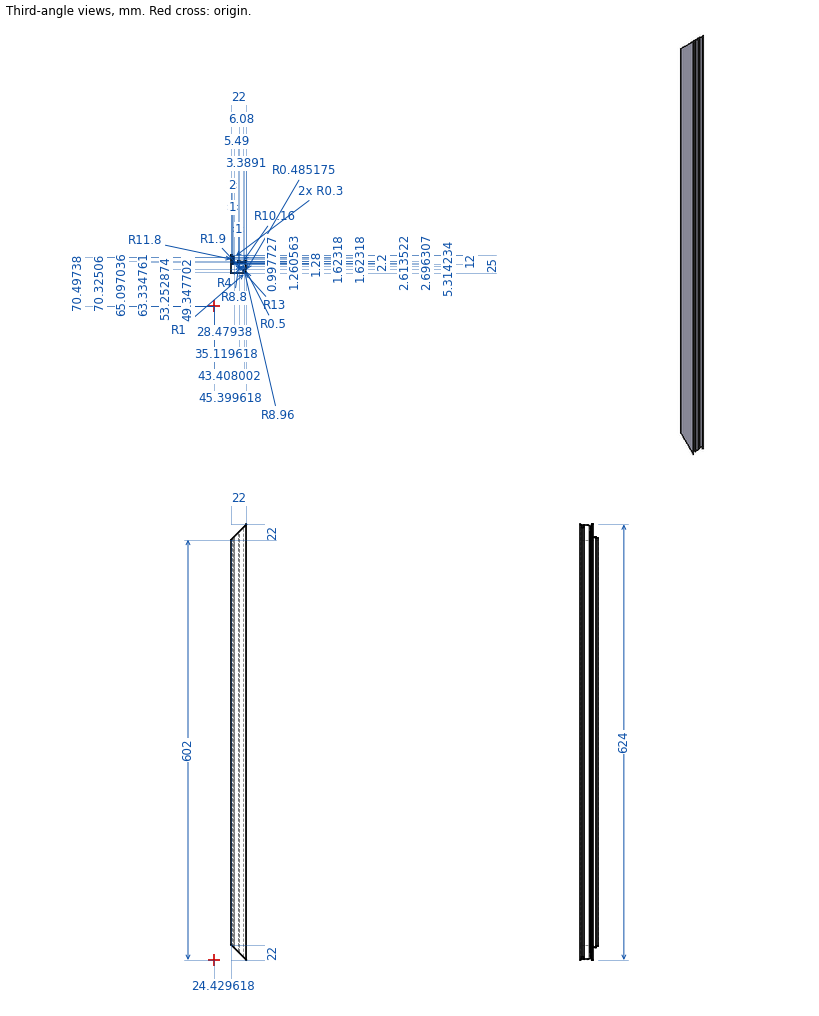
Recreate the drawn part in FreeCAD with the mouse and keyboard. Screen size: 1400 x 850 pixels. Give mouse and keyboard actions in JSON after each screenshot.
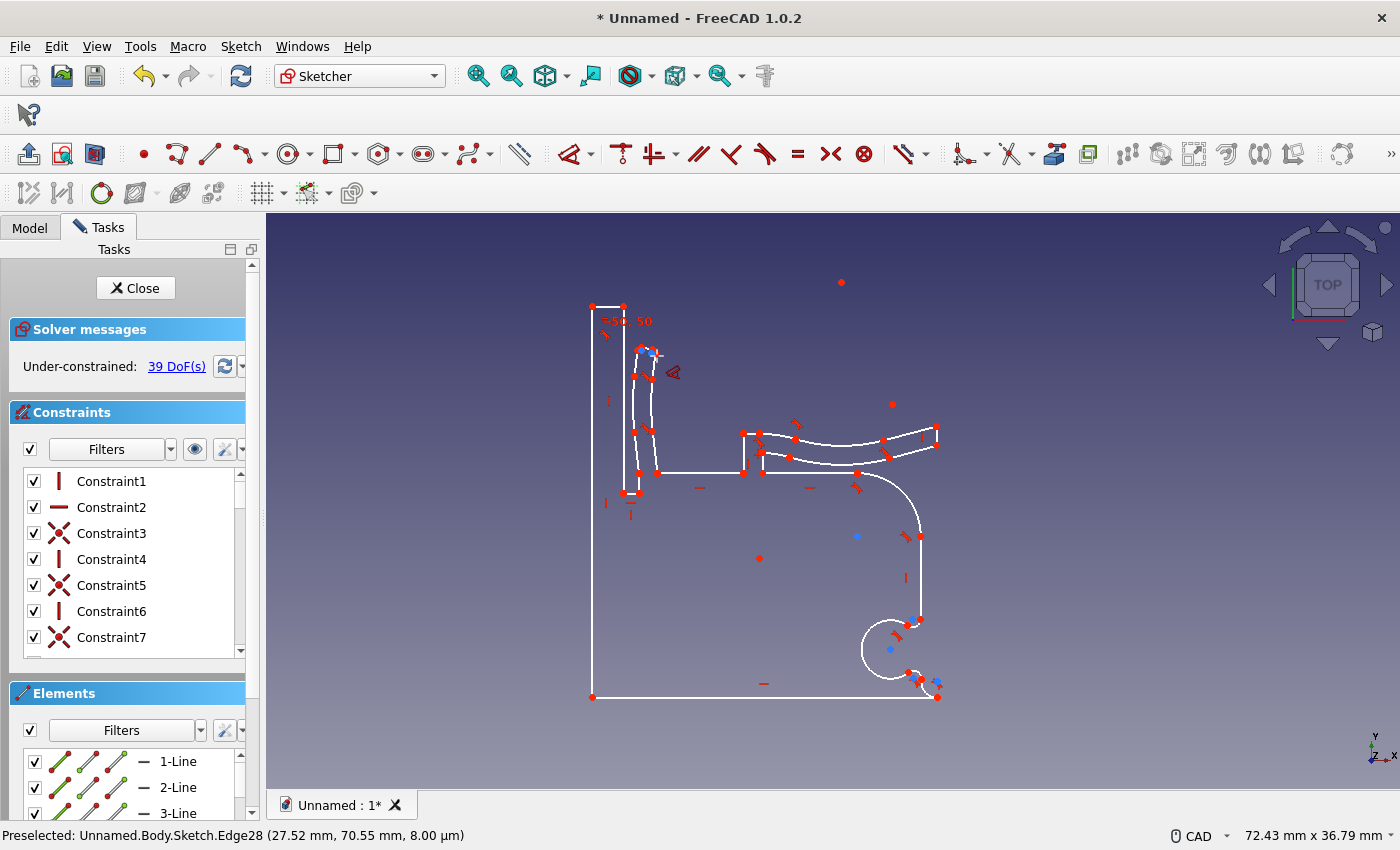
{"action": "left_click", "coordinate": [914, 508]}
{"action": "left_click", "coordinate": [943, 494]}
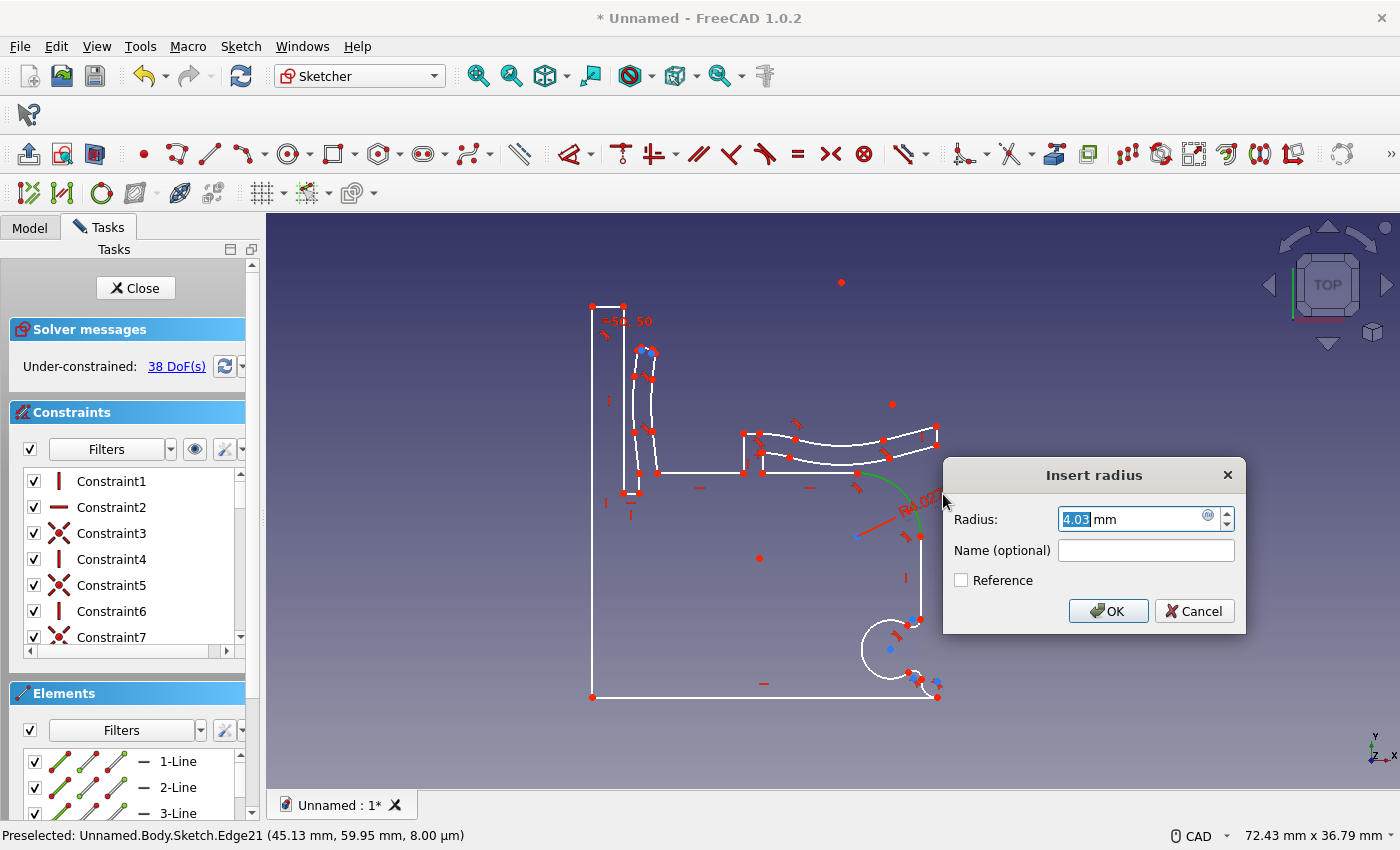
{"action": "type", "text": "4"}
{"action": "key", "text": "Return"}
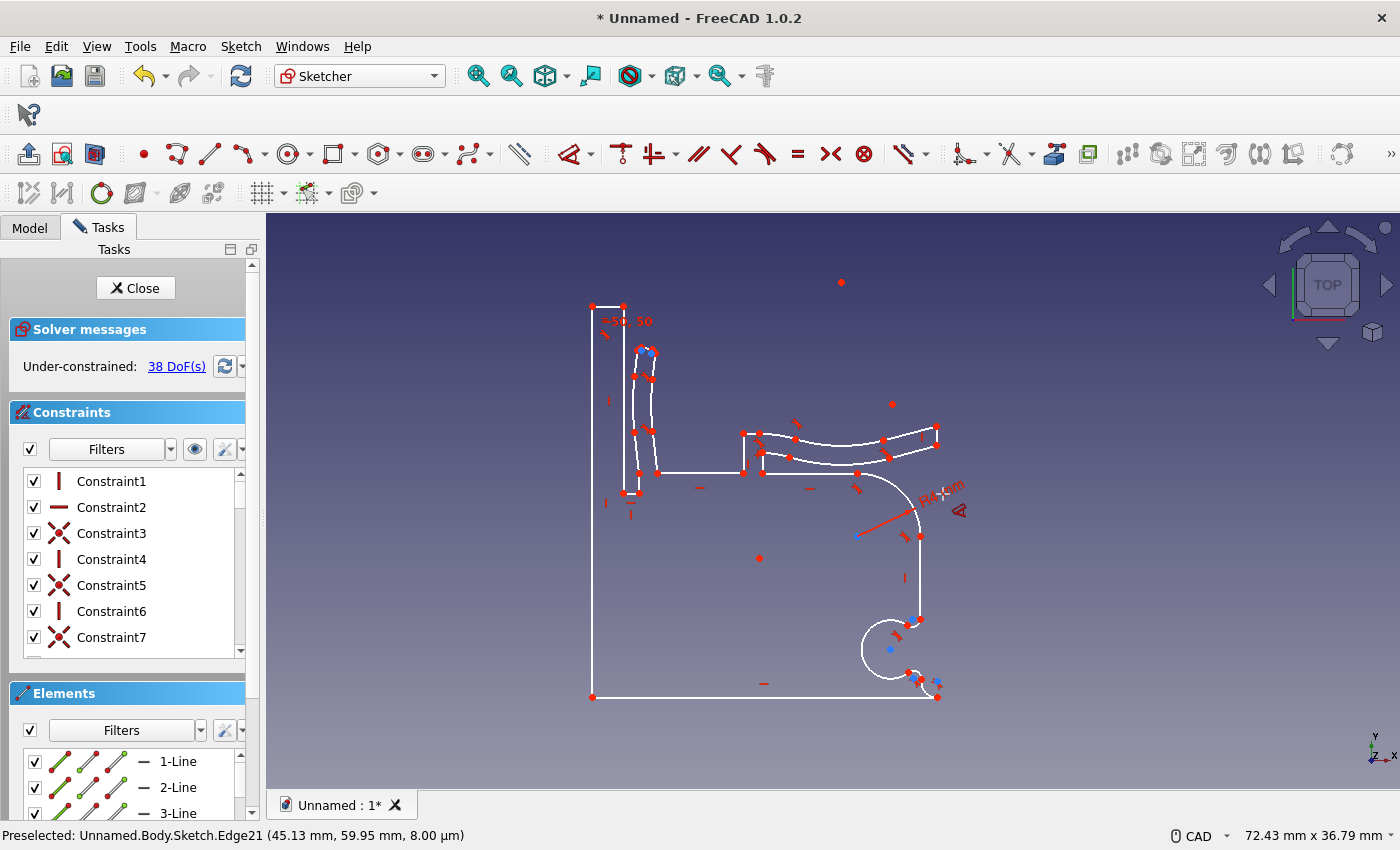
{"action": "left_click", "coordinate": [776, 454]}
{"action": "left_click", "coordinate": [781, 422]}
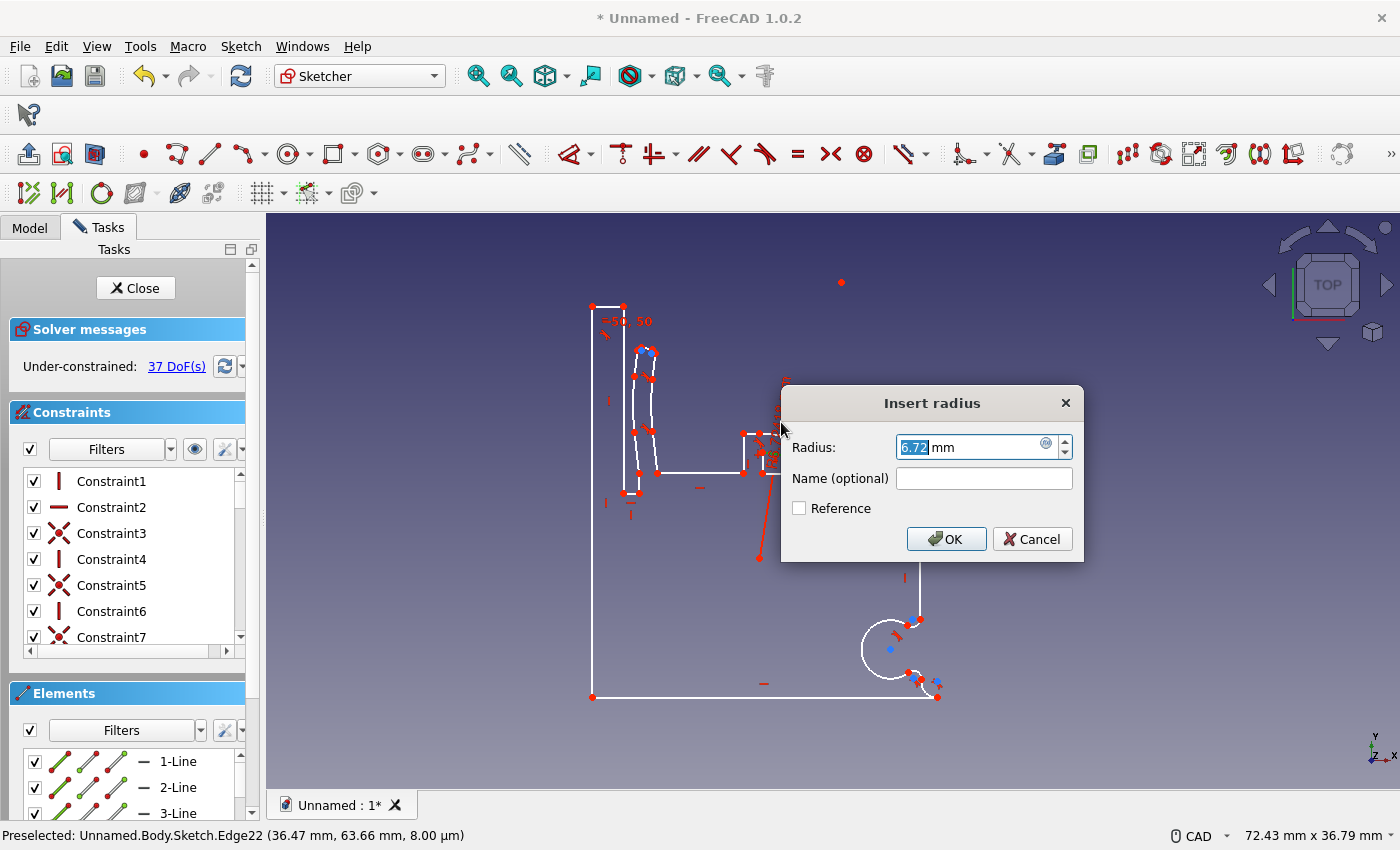
{"action": "type", "text": "8.8"}
{"action": "key", "text": "Return"}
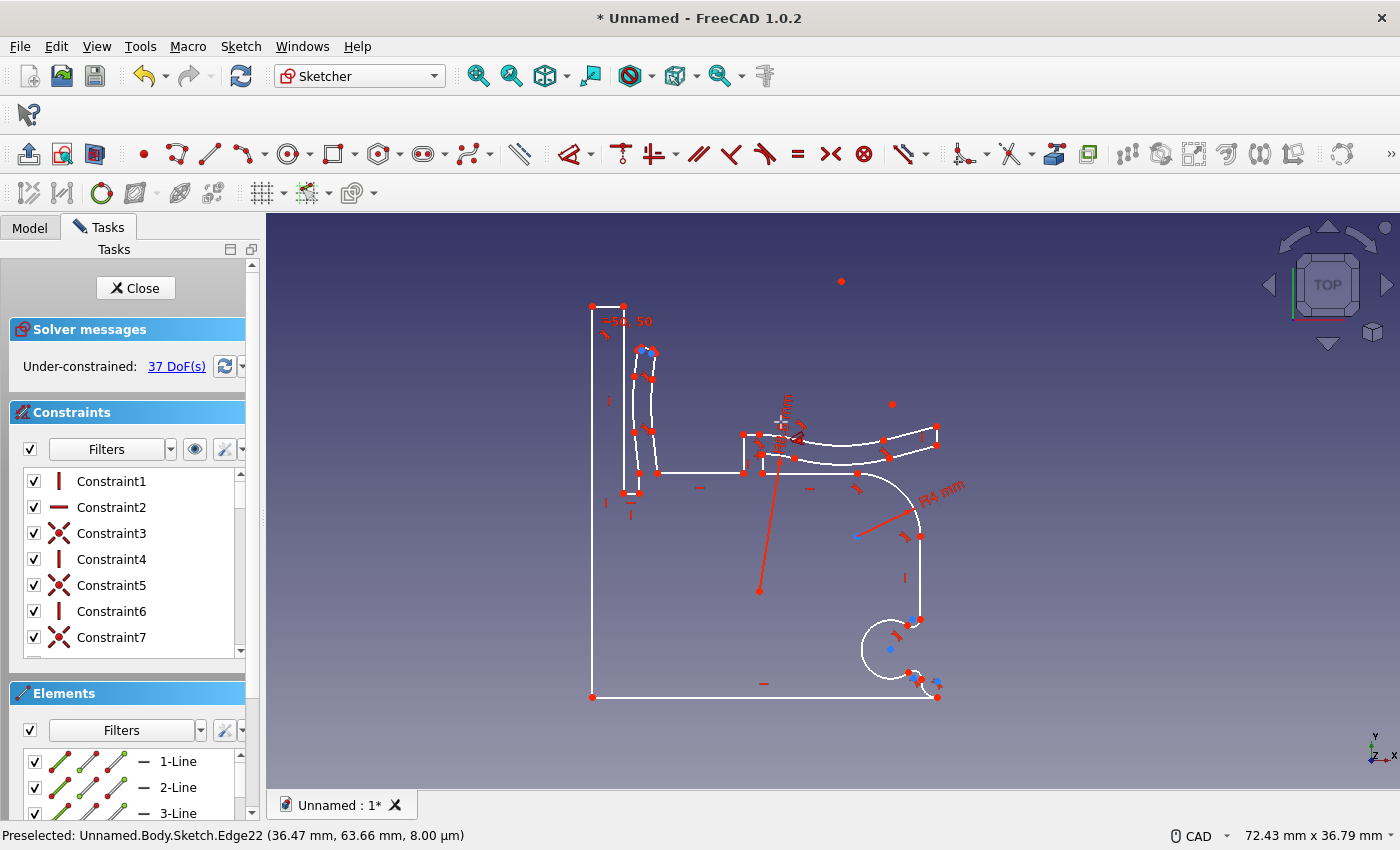
{"action": "scroll", "coordinate": [823, 464], "scroll_direction": "up", "scroll_amount": 2}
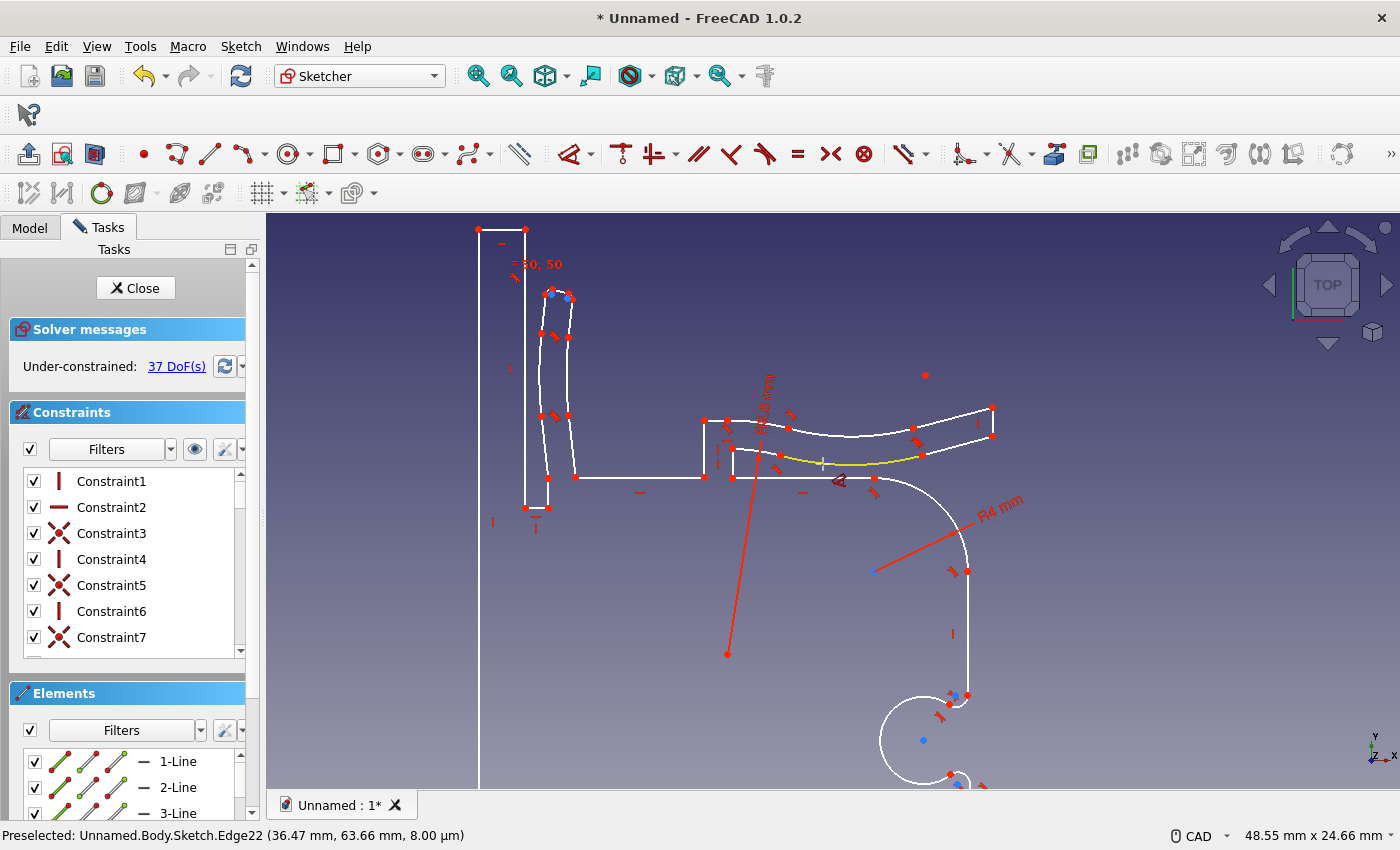
{"action": "left_click", "coordinate": [823, 464]}
{"action": "left_click", "coordinate": [820, 496]}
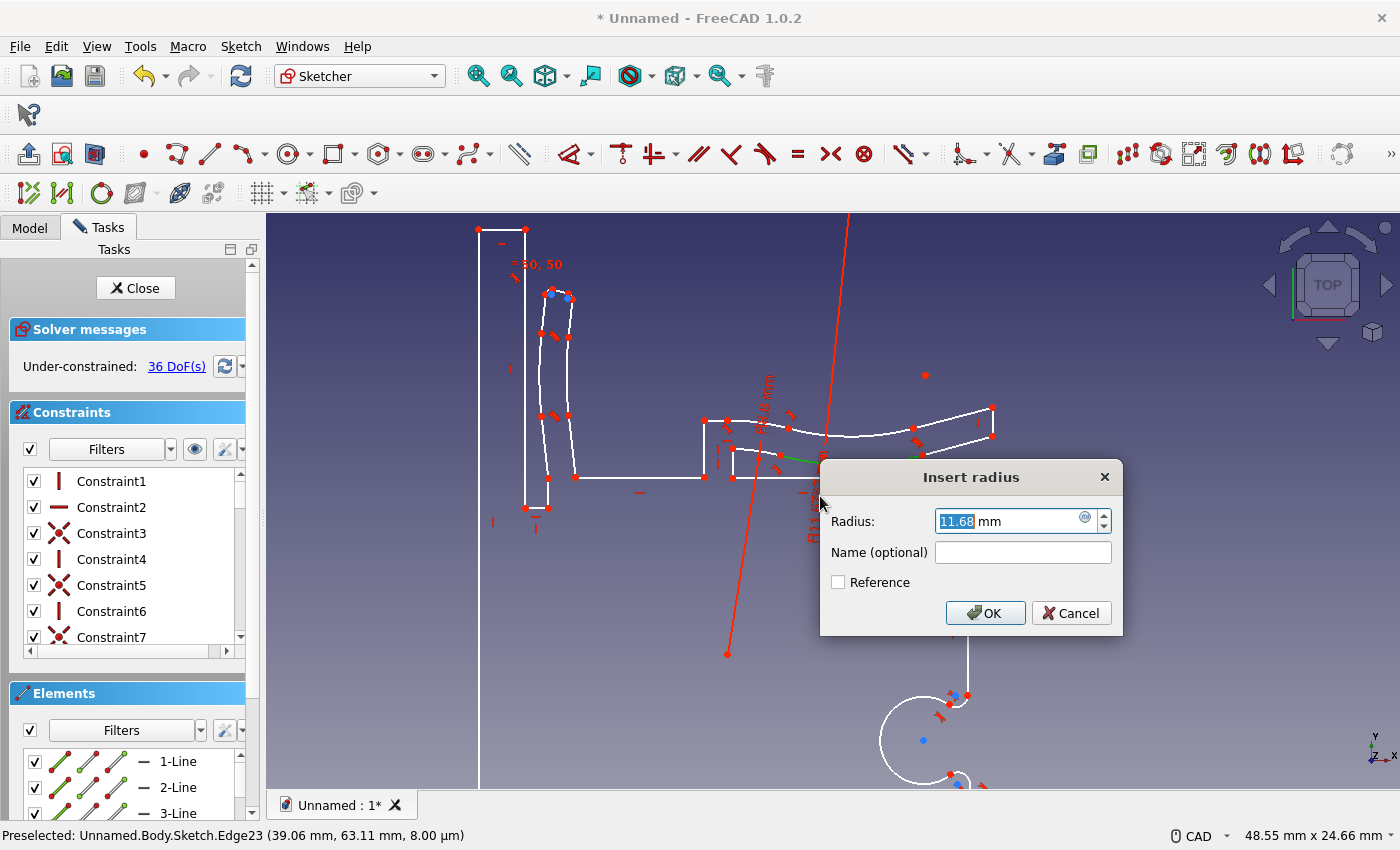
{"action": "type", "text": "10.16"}
{"action": "key", "text": "Return"}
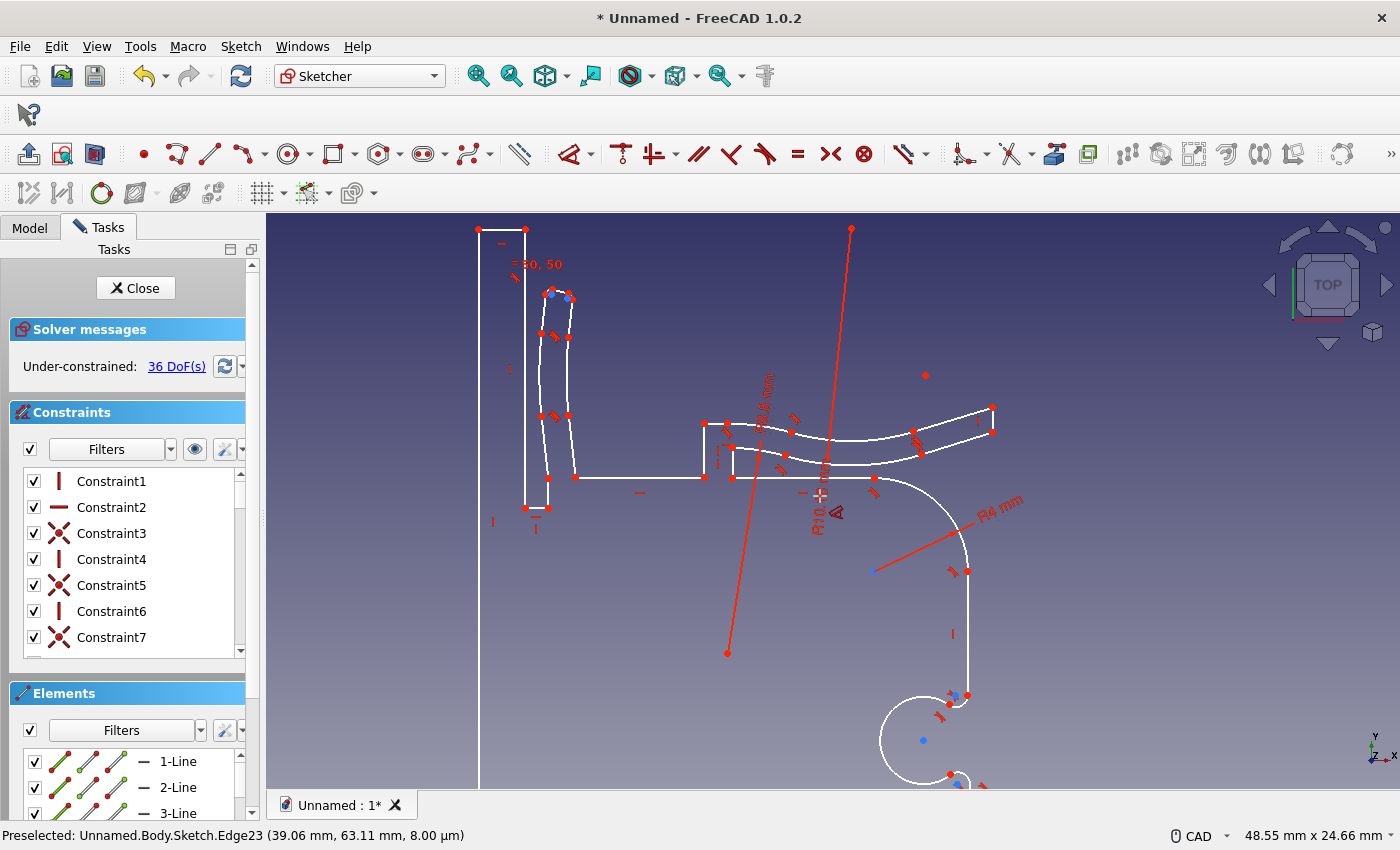
{"action": "left_click", "coordinate": [828, 440]}
{"action": "left_click", "coordinate": [632, 337]}